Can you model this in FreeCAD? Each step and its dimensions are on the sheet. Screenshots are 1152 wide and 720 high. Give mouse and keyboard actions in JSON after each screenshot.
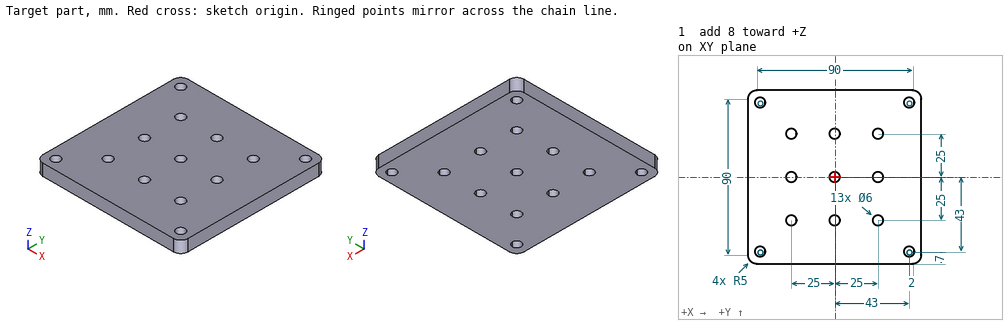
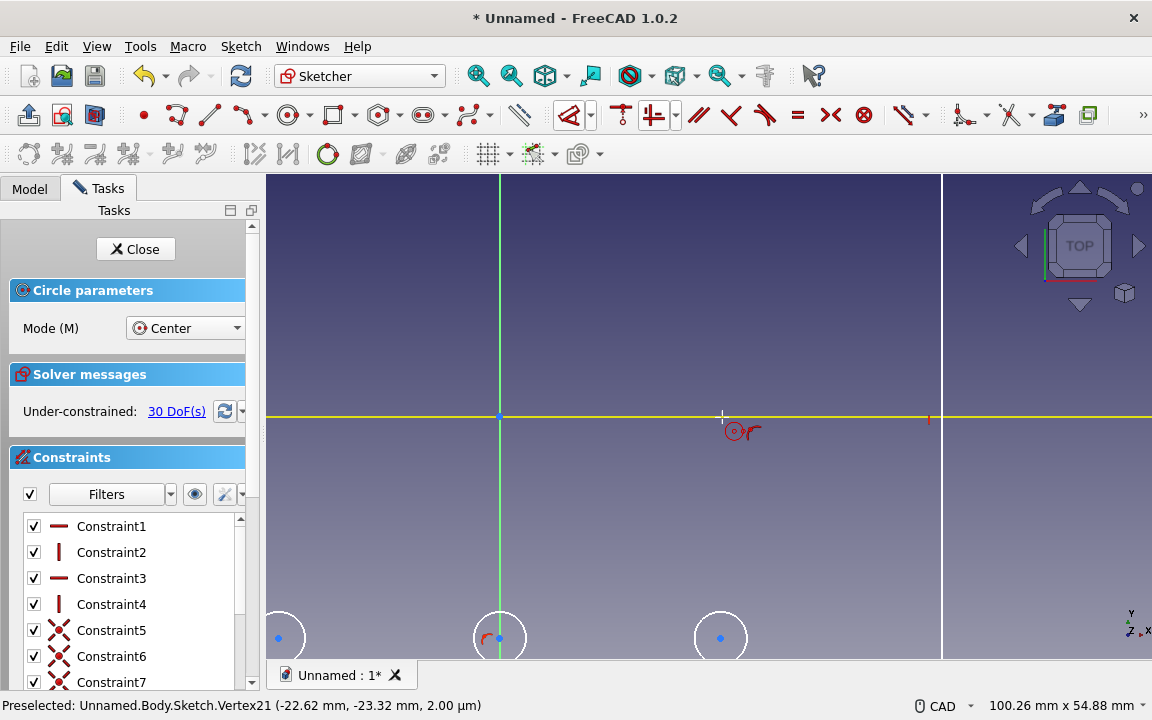
{"action": "left_click", "coordinate": [721, 417]}
{"action": "left_click", "coordinate": [740, 398]}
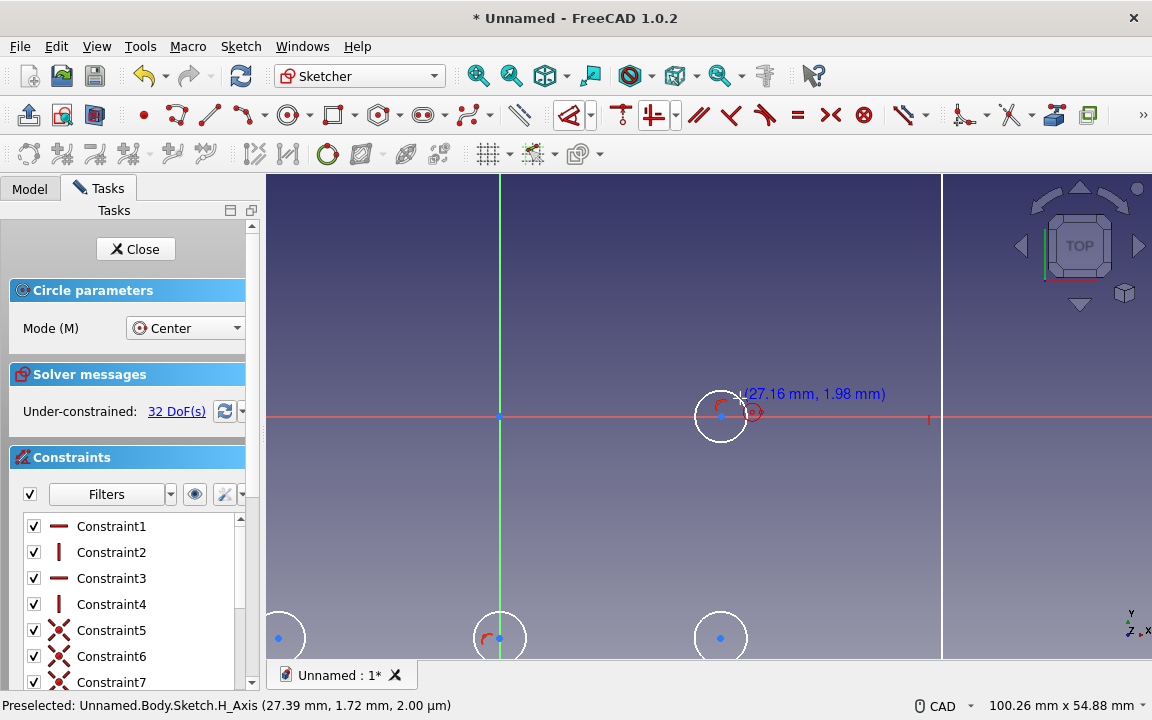
{"action": "scroll", "coordinate": [722, 416], "scroll_direction": "down", "scroll_amount": 5}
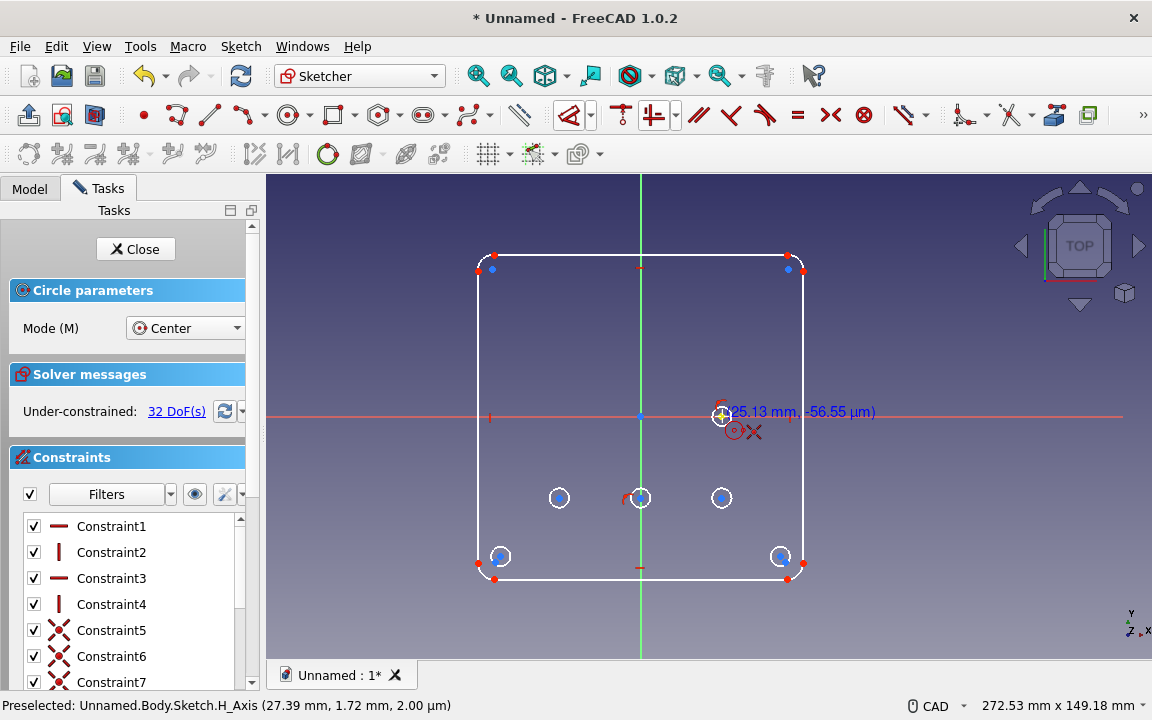
{"action": "scroll", "coordinate": [722, 335], "scroll_direction": "up", "scroll_amount": 5}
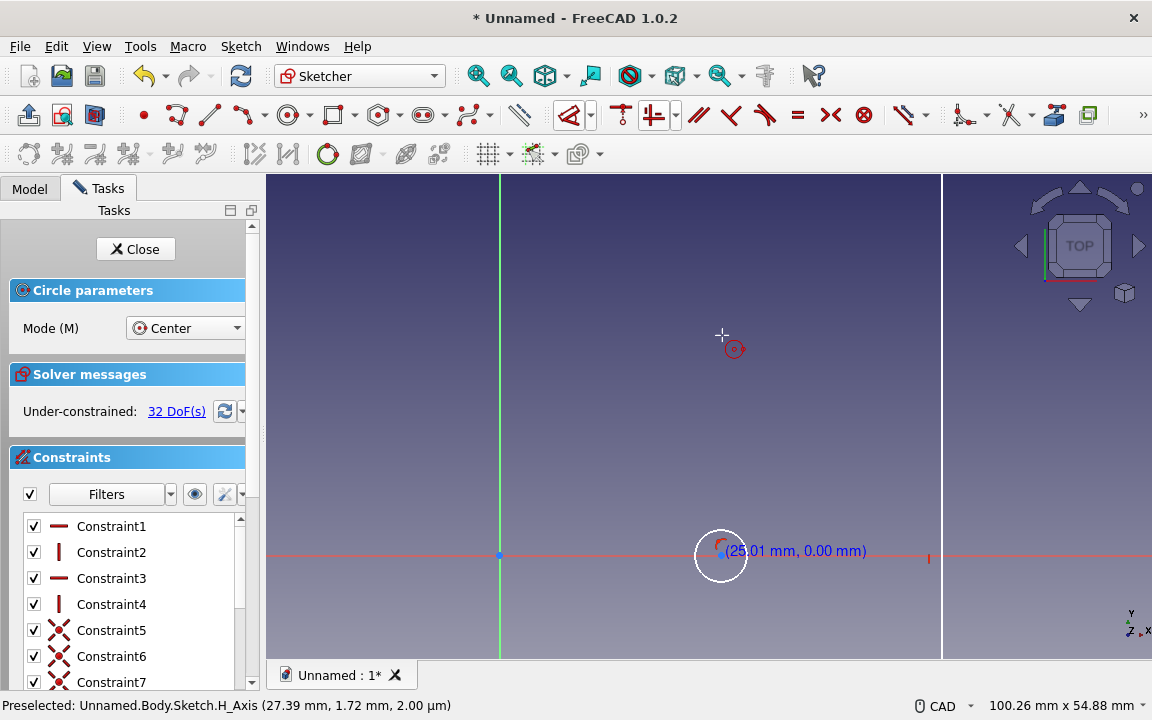
{"action": "left_click", "coordinate": [721, 335]}
{"action": "left_click", "coordinate": [740, 316]}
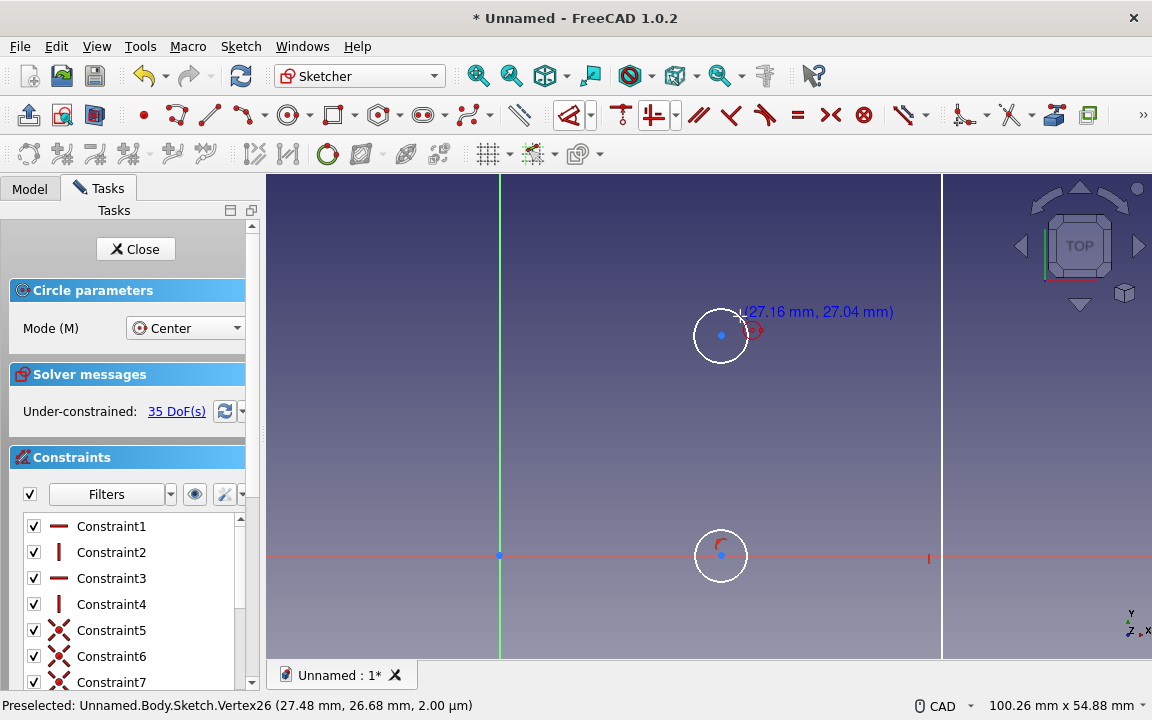
{"action": "scroll", "coordinate": [722, 335], "scroll_direction": "down", "scroll_amount": 5}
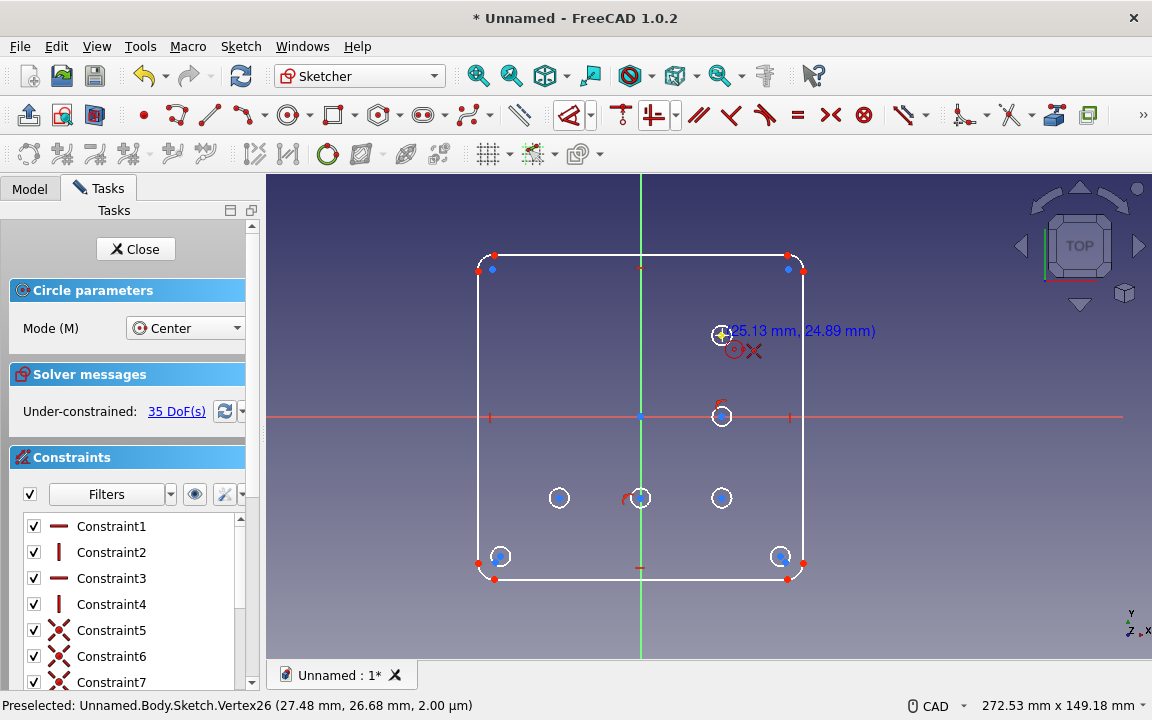
{"action": "scroll", "coordinate": [780, 277], "scroll_direction": "up", "scroll_amount": 5}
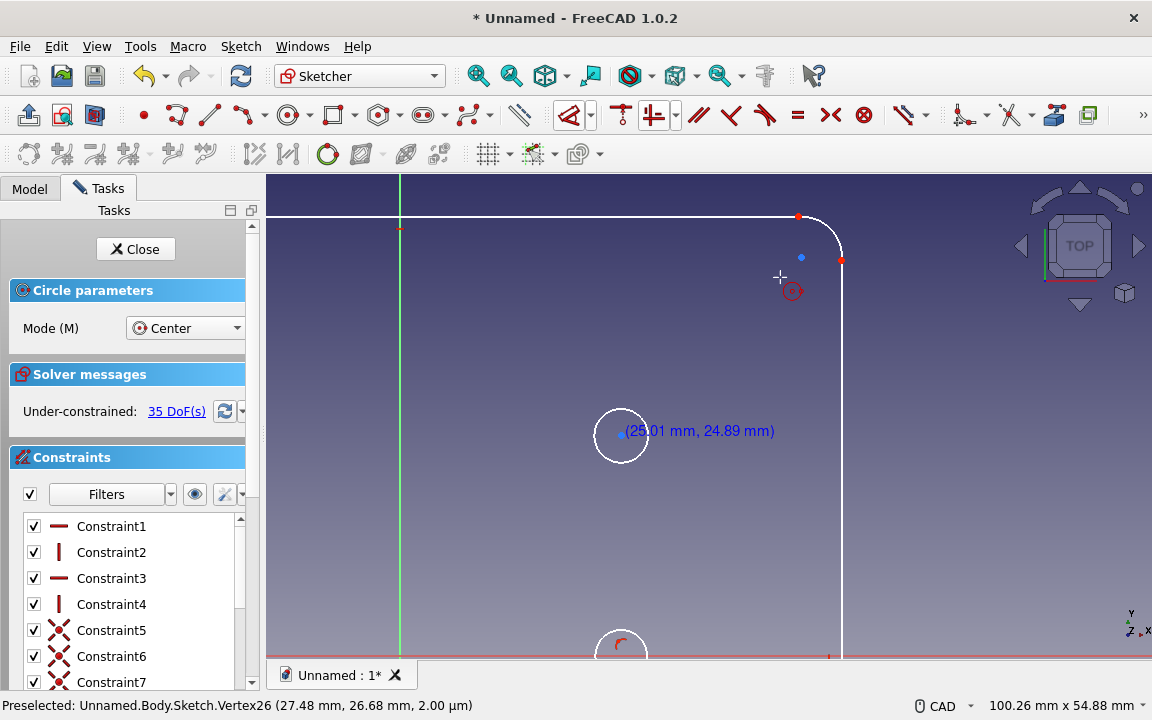
{"action": "left_click", "coordinate": [780, 276]}
{"action": "left_click", "coordinate": [761, 257]}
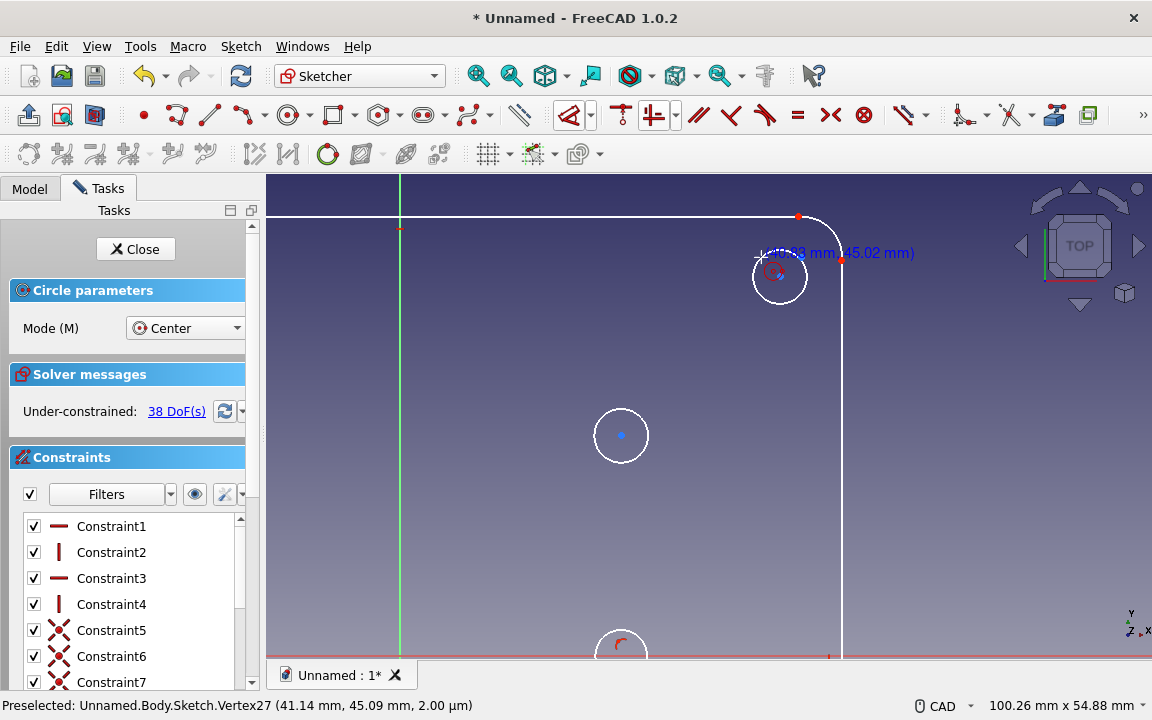
{"action": "scroll", "coordinate": [780, 277], "scroll_direction": "down", "scroll_amount": 5}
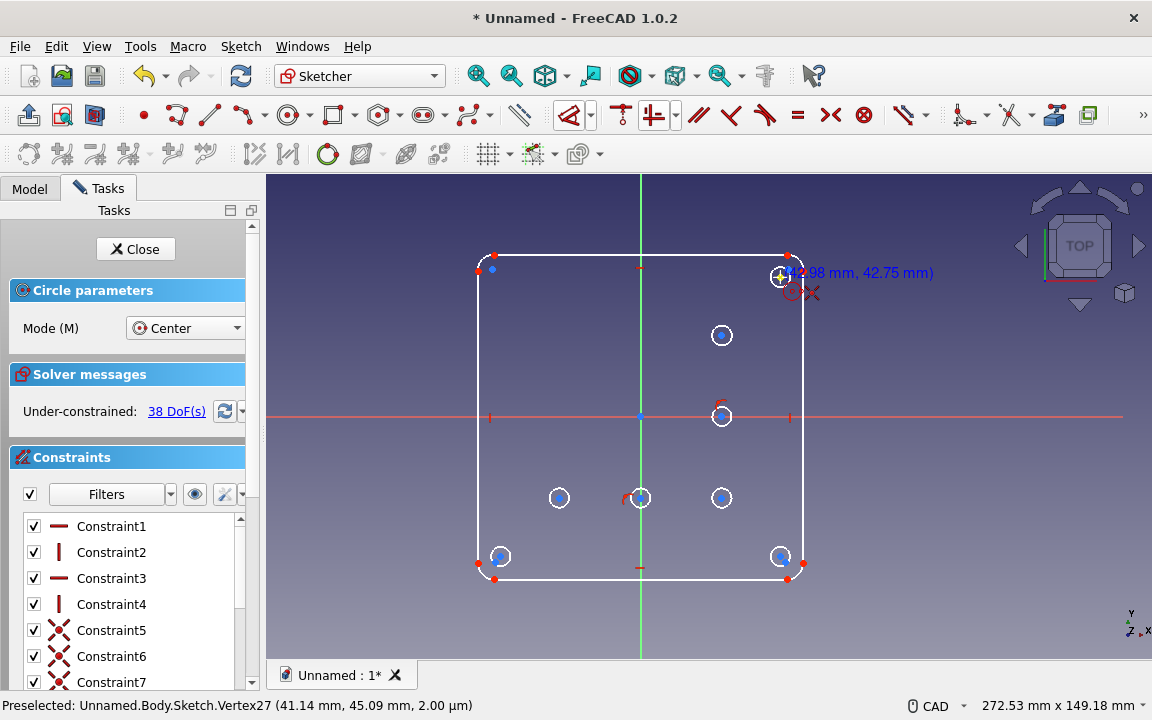
{"action": "scroll", "coordinate": [641, 417], "scroll_direction": "up", "scroll_amount": 5}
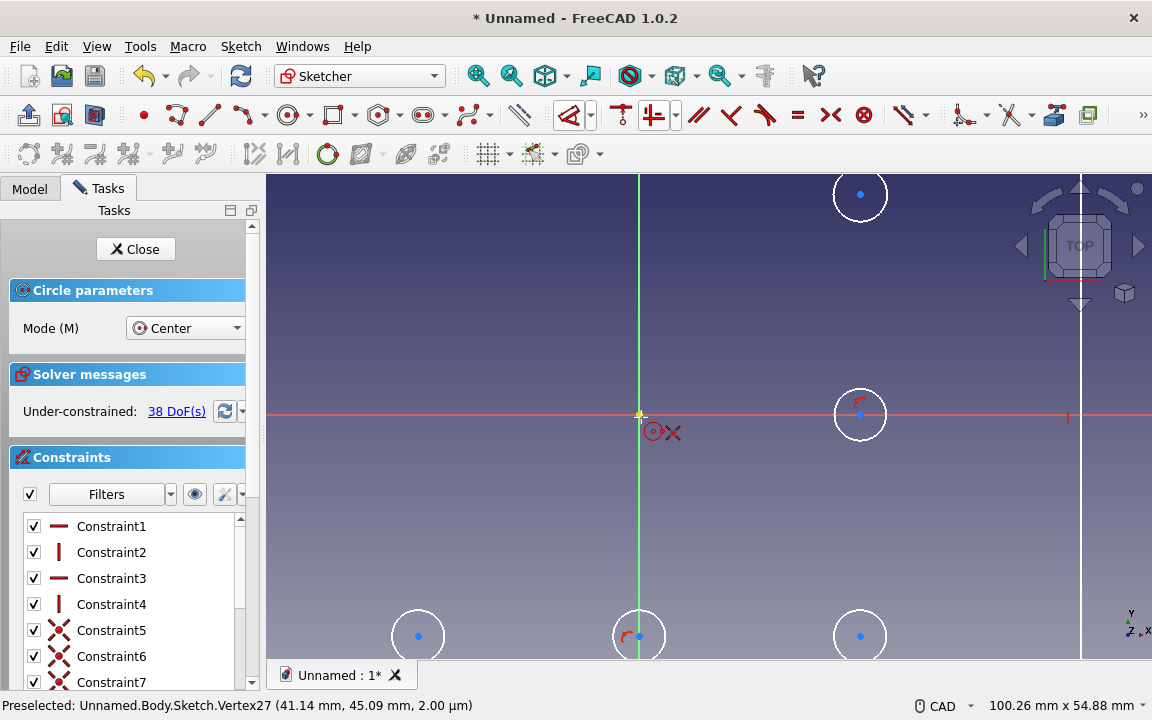
{"action": "left_click", "coordinate": [639, 415]}
{"action": "left_click", "coordinate": [658, 396]}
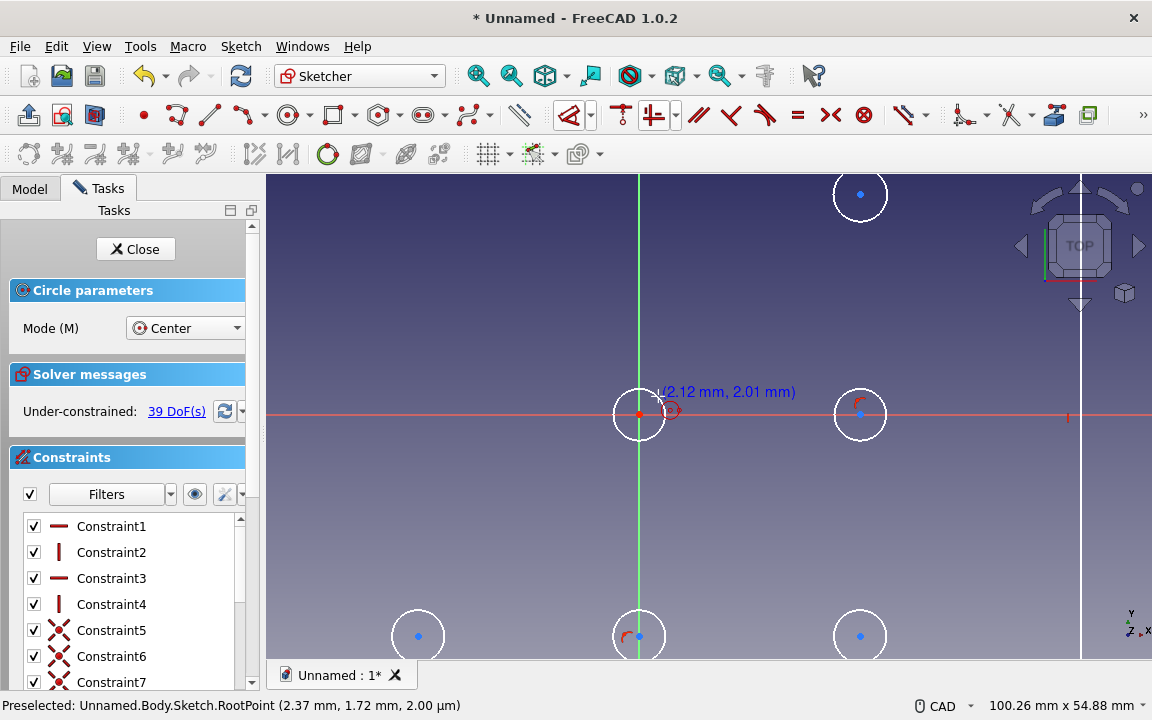
{"action": "left_click", "coordinate": [418, 415]}
{"action": "left_click", "coordinate": [437, 396]}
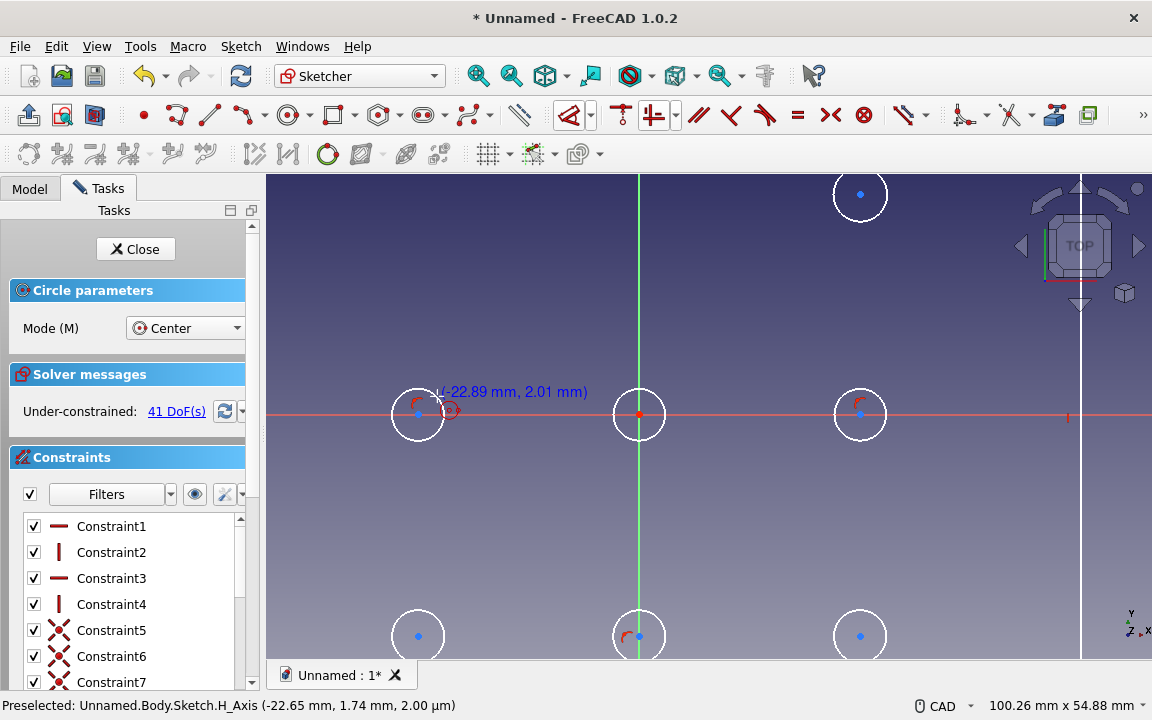
{"action": "scroll", "coordinate": [641, 418], "scroll_direction": "down", "scroll_amount": 5}